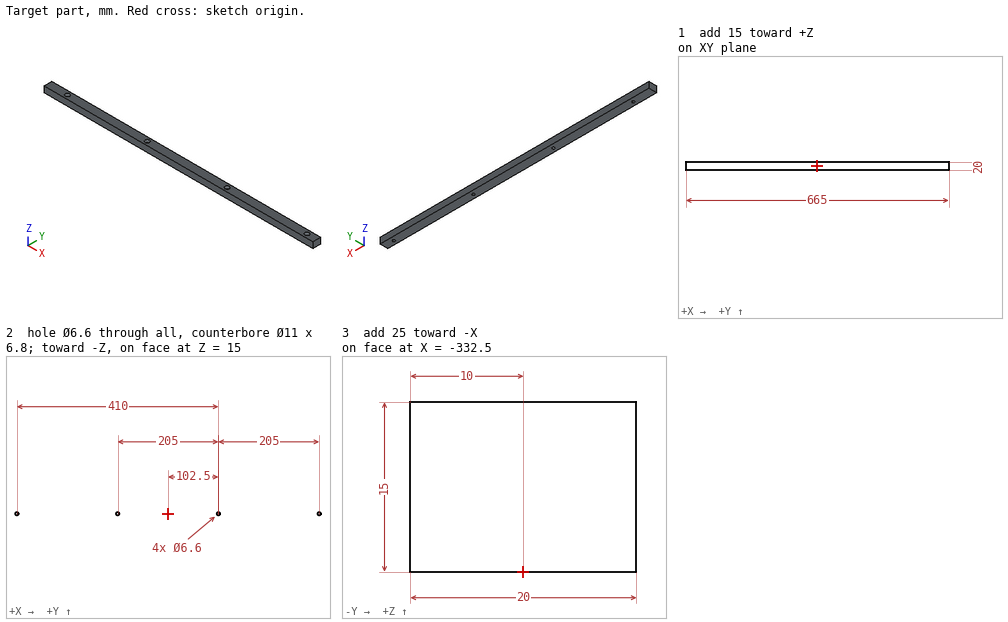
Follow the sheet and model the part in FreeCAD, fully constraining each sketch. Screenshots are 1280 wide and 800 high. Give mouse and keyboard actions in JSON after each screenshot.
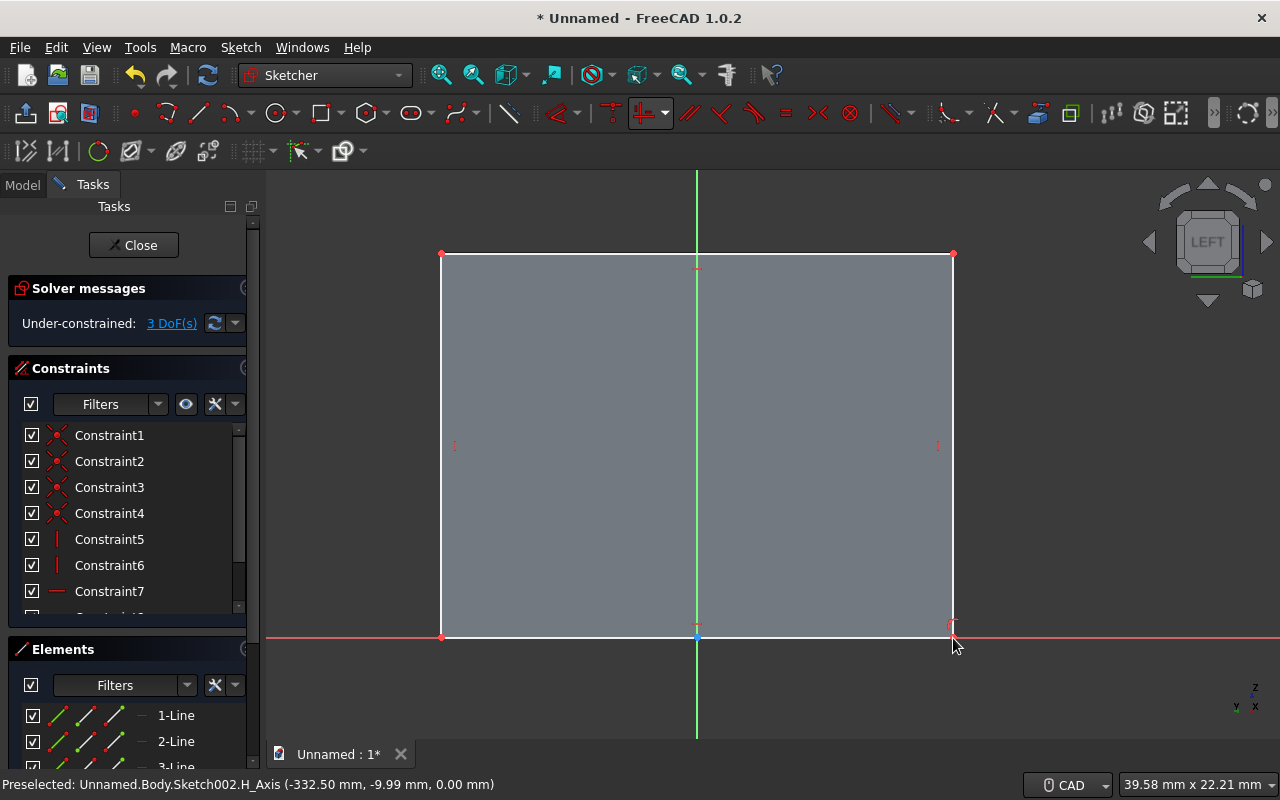
{"action": "left_click", "coordinate": [441, 369]}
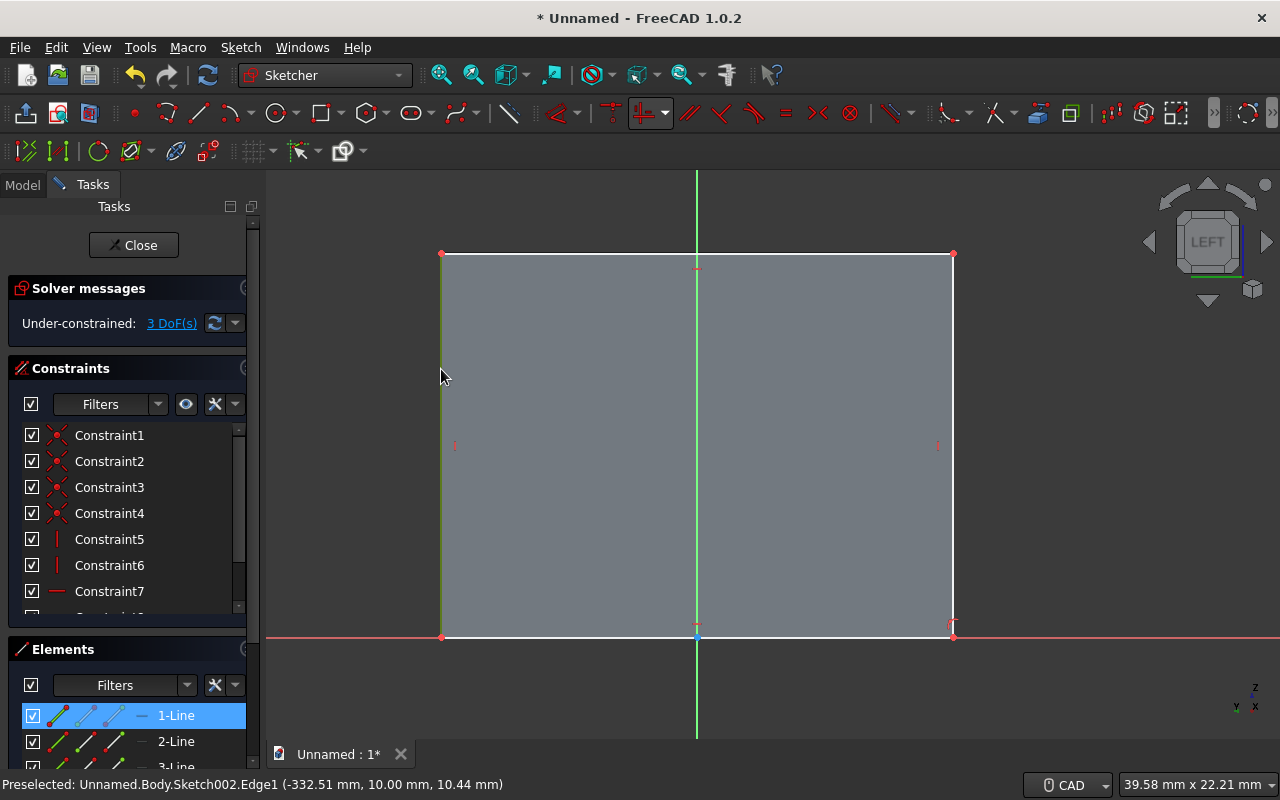
{"action": "key", "text": "i"}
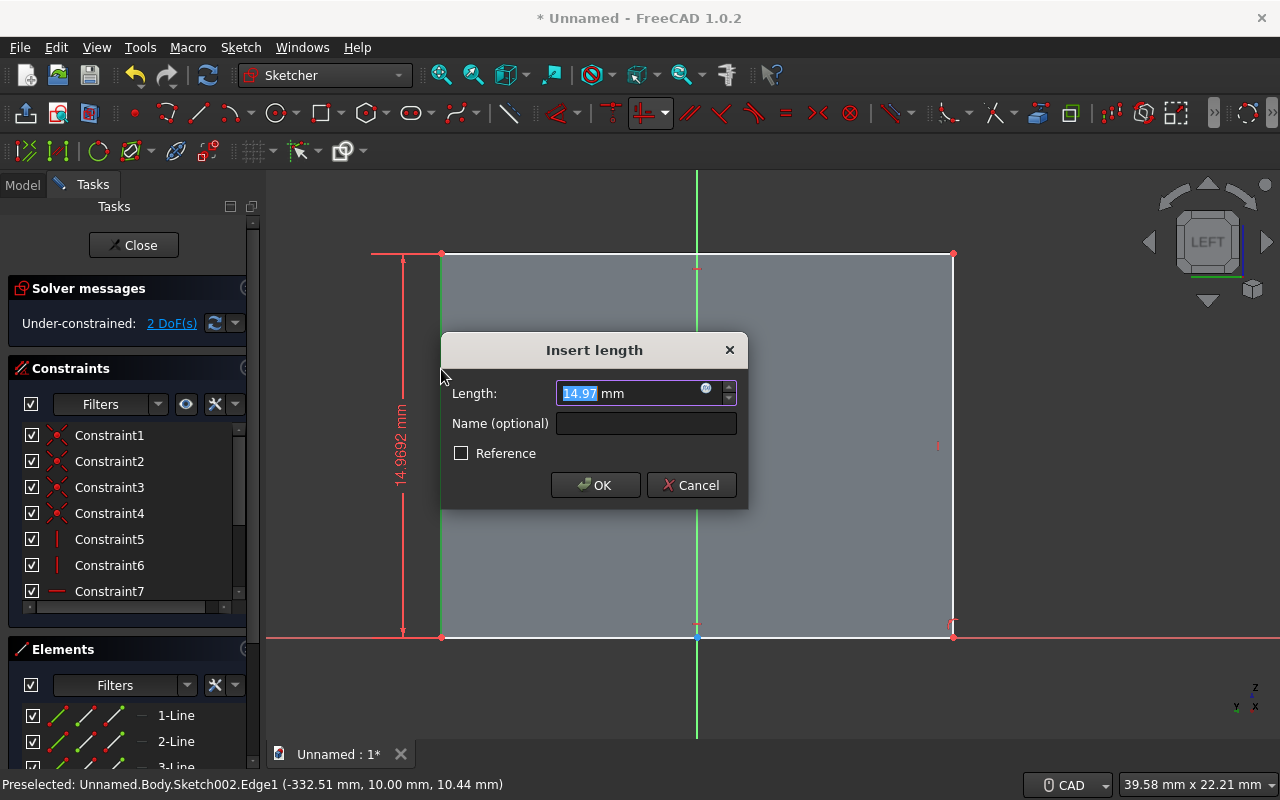
{"action": "type", "text": "15"}
{"action": "key", "text": "Return"}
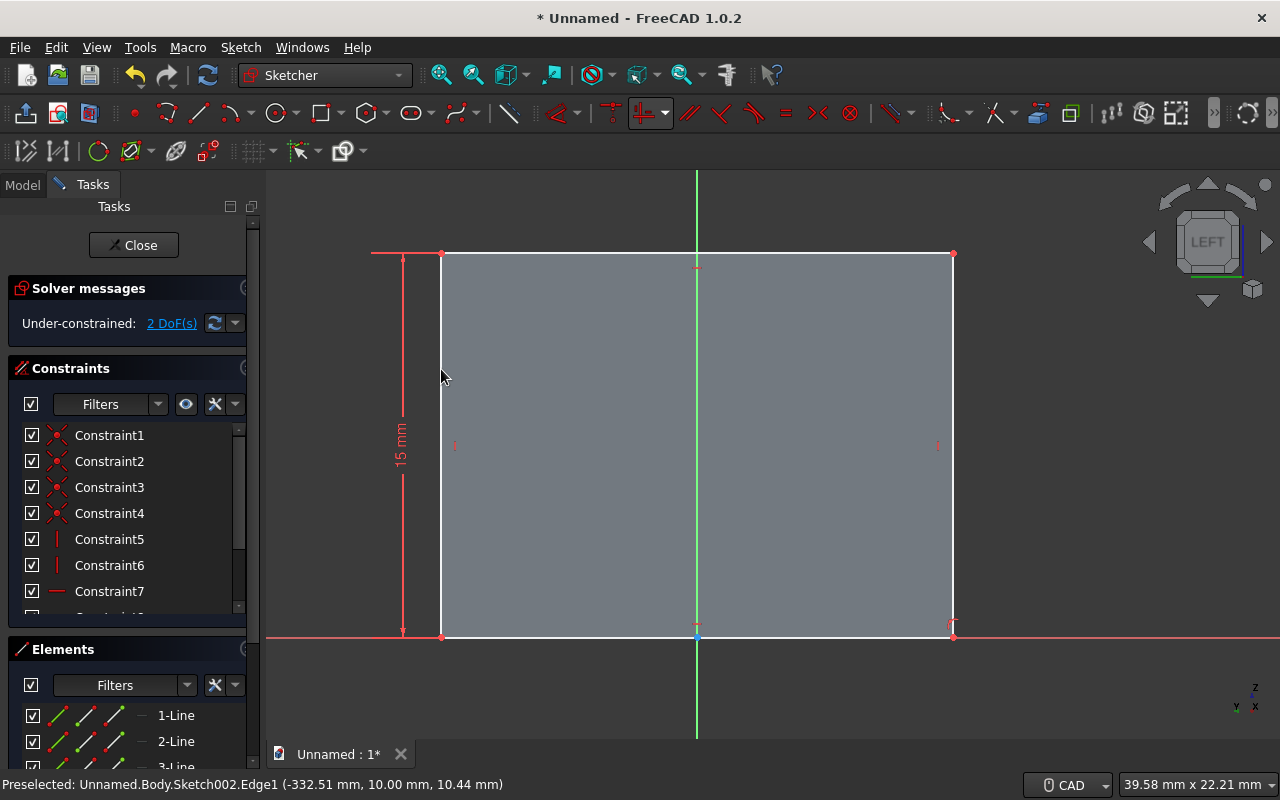
{"action": "left_click", "coordinate": [595, 638]}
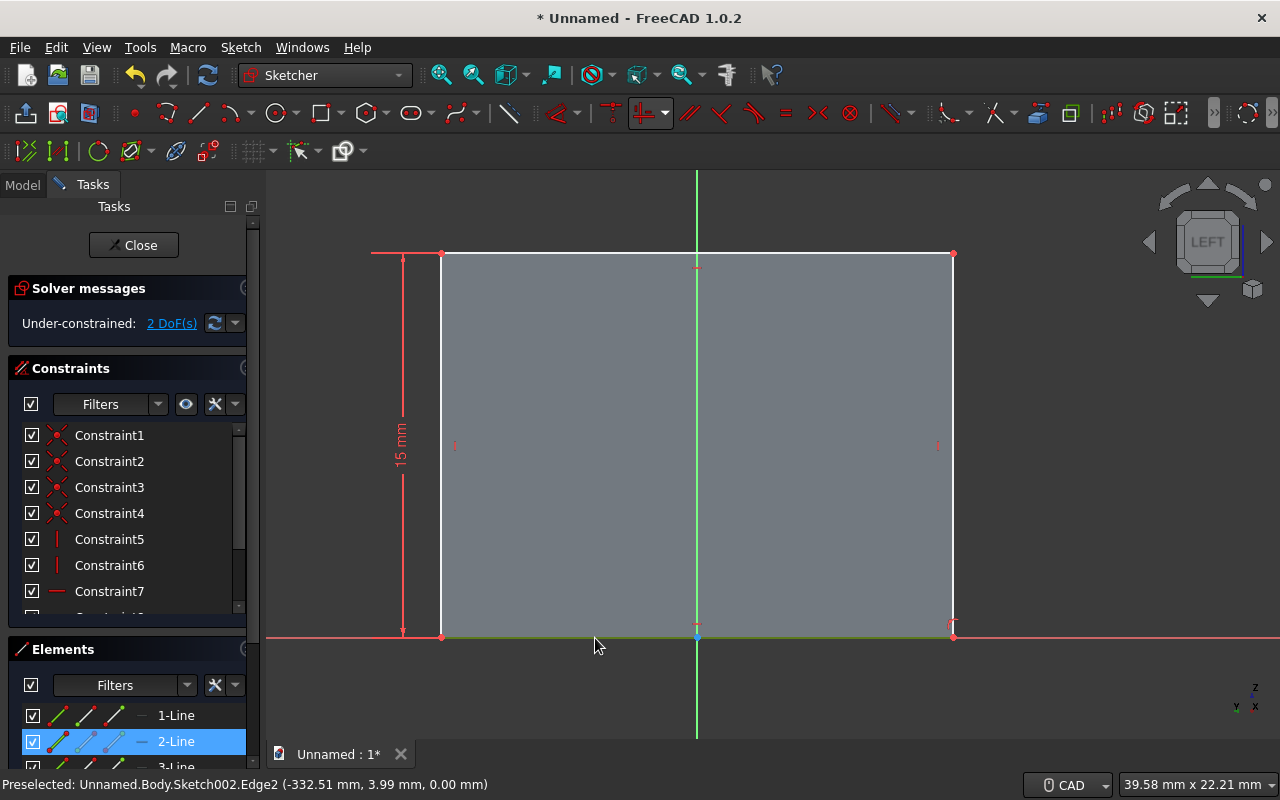
{"action": "key", "text": "l"}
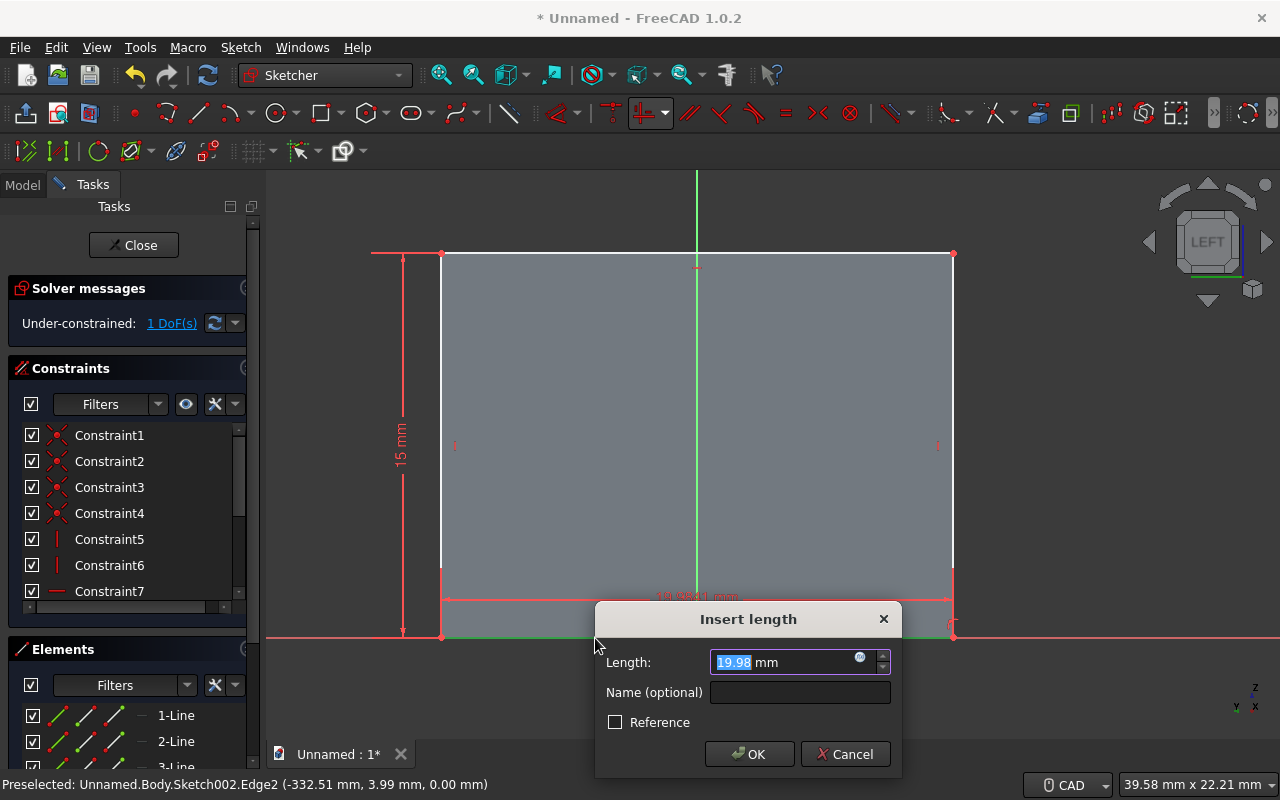
{"action": "type", "text": "20"}
{"action": "key", "text": "Return"}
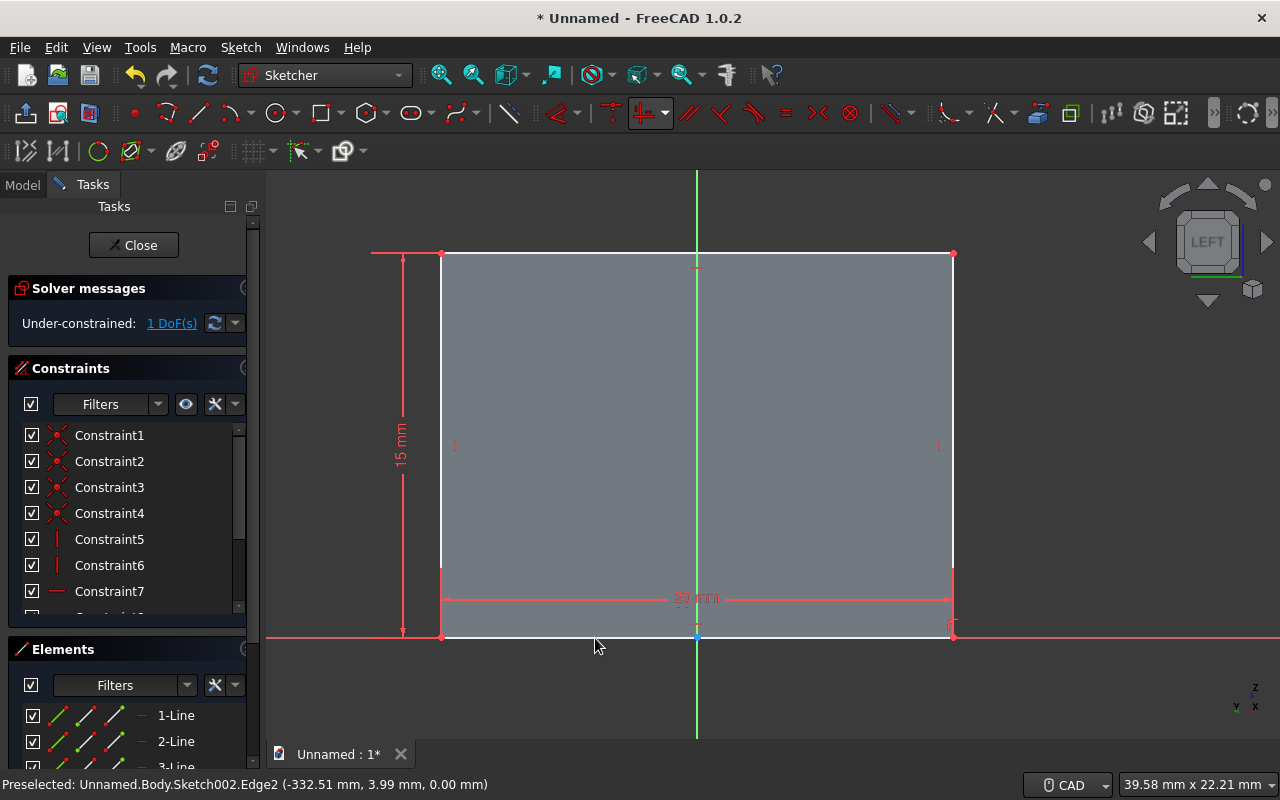
{"action": "left_click", "coordinate": [441, 253]}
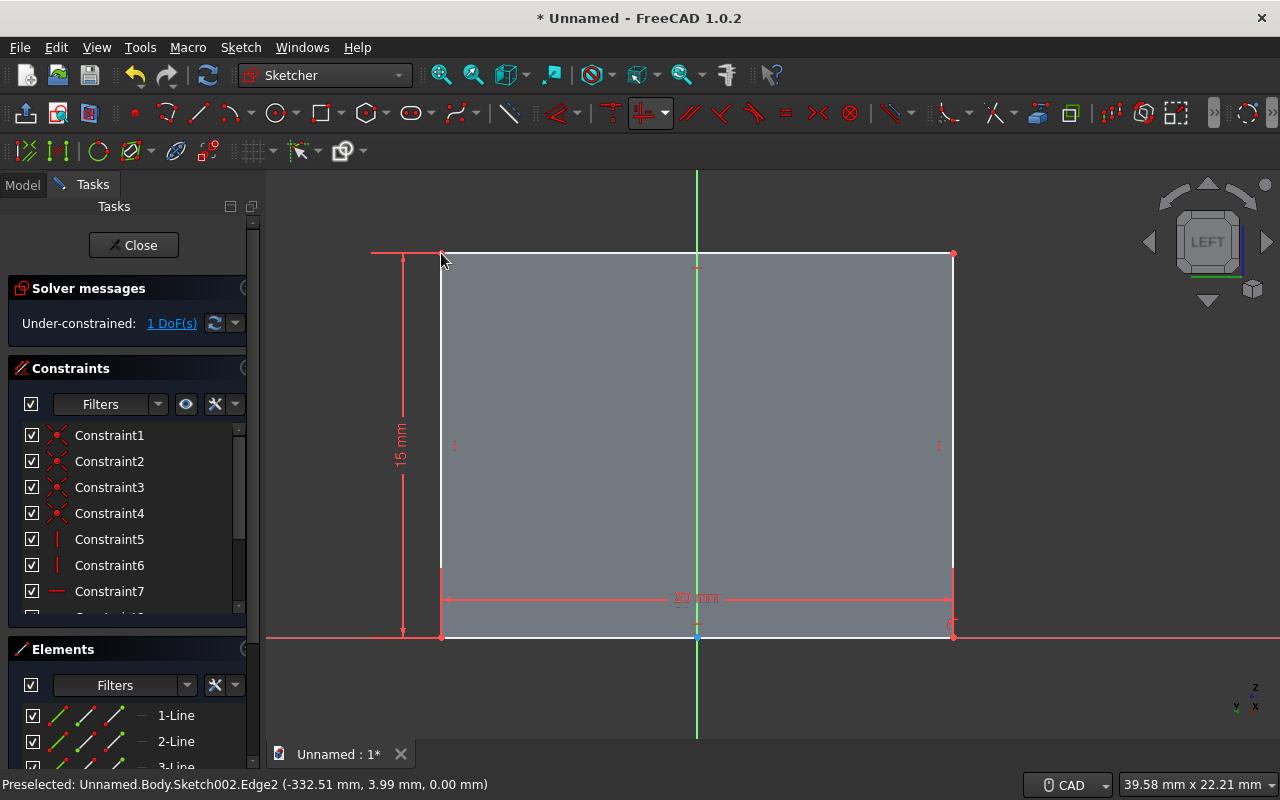
{"action": "key", "text": "l"}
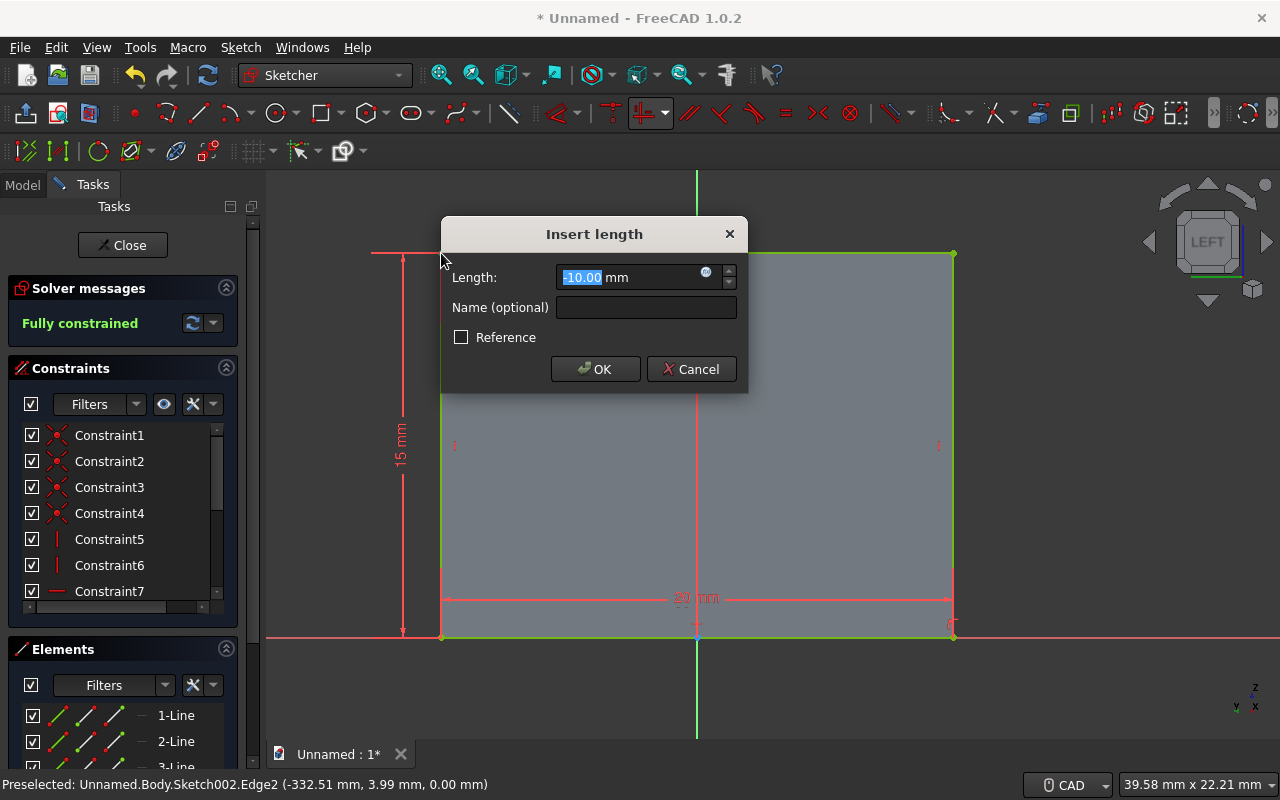
{"action": "type", "text": "-10"}
{"action": "key", "text": "Return"}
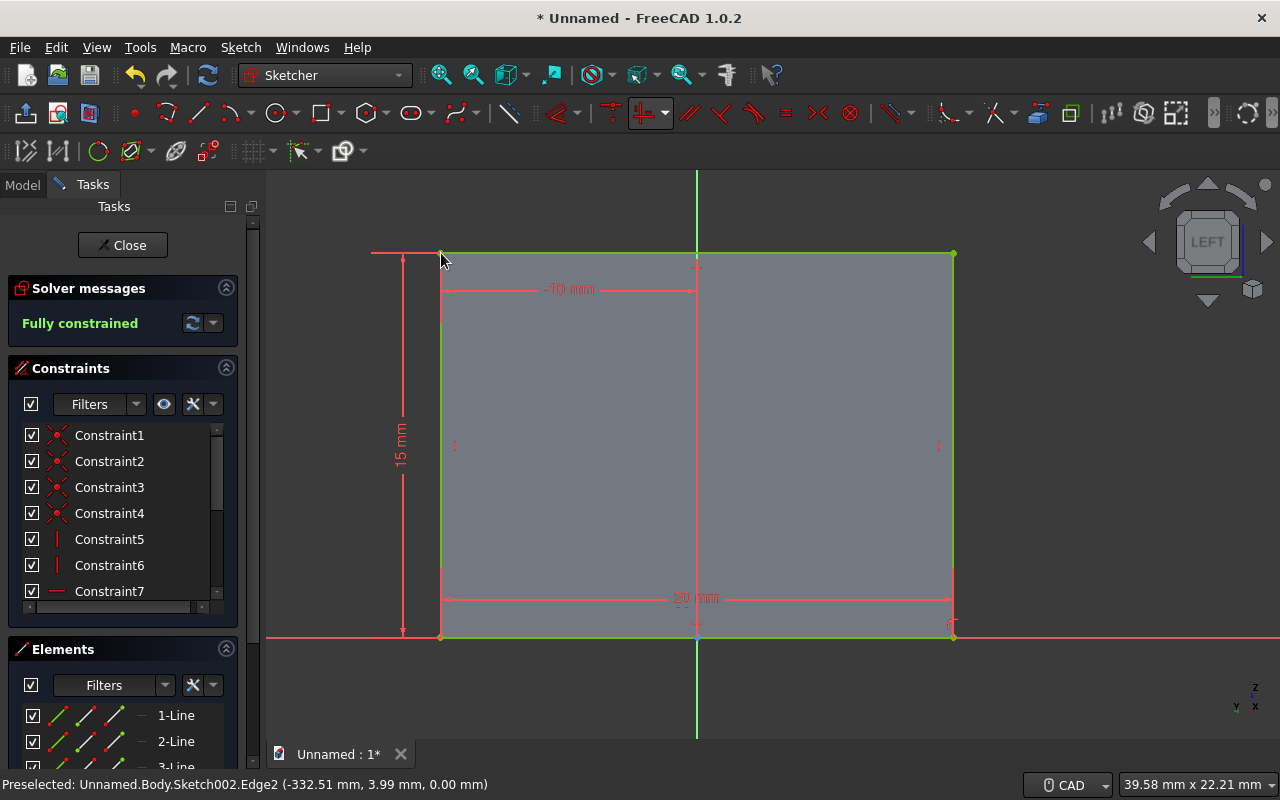
{"action": "left_click", "coordinate": [123, 245]}